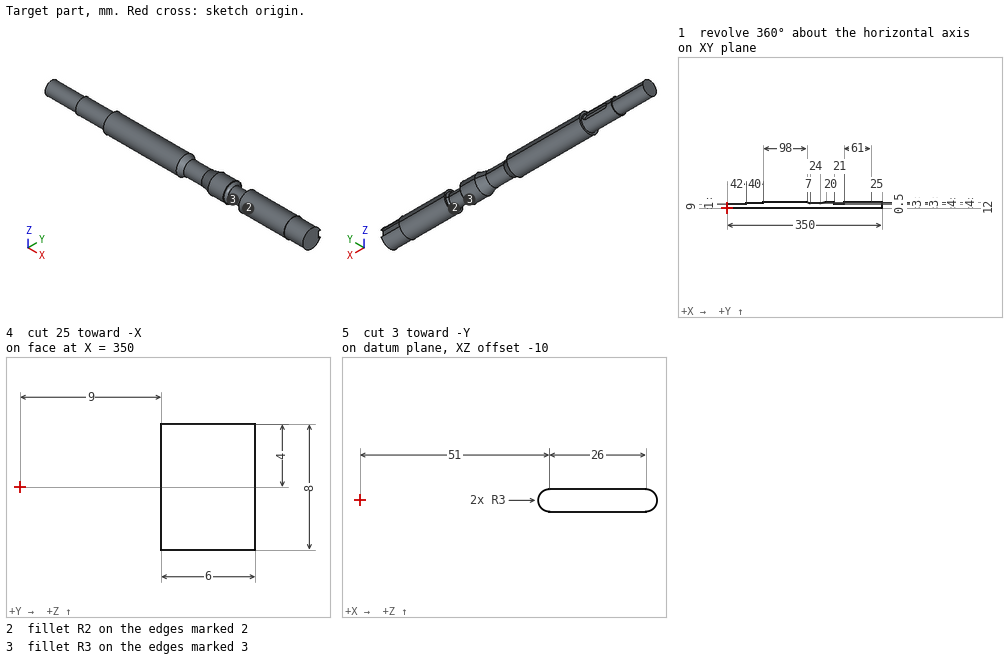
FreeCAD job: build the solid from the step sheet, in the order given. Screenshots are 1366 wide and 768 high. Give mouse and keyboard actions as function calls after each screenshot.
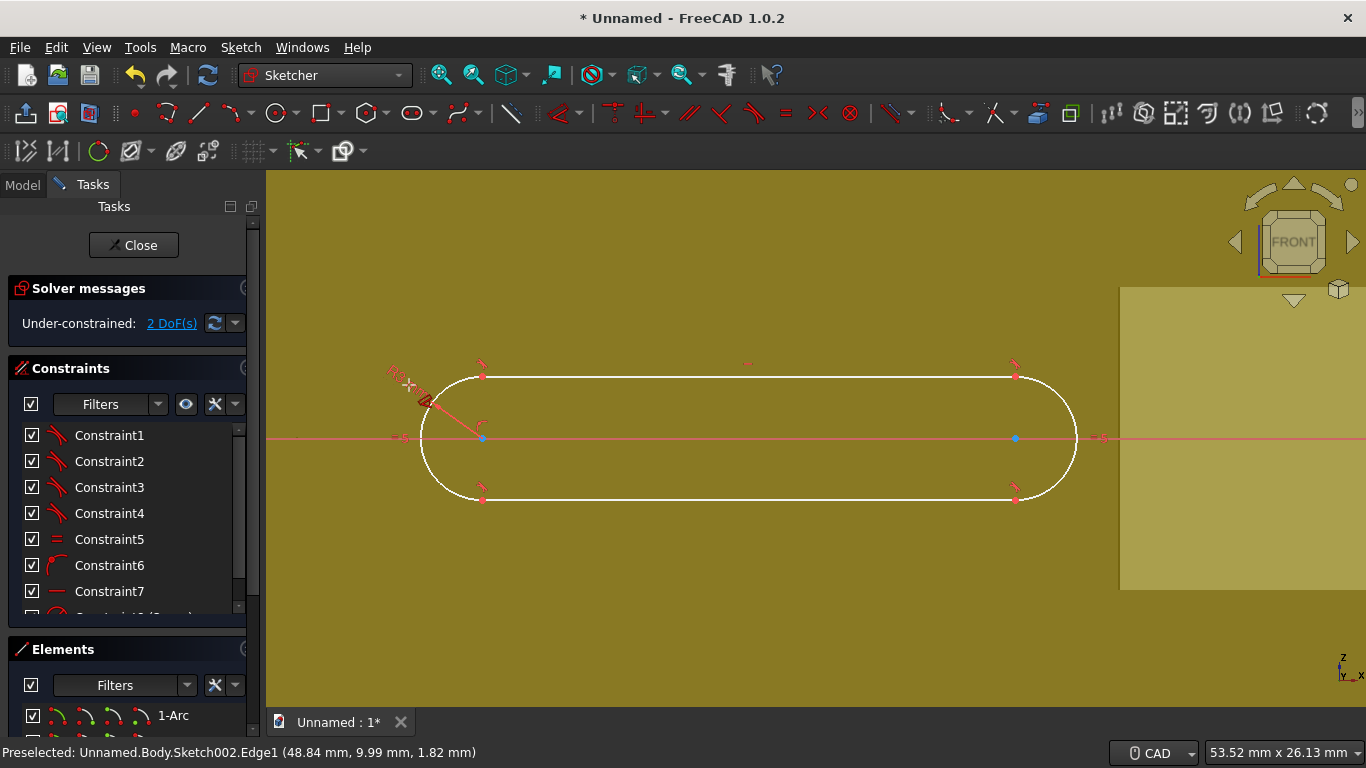
click(642, 377)
click(749, 343)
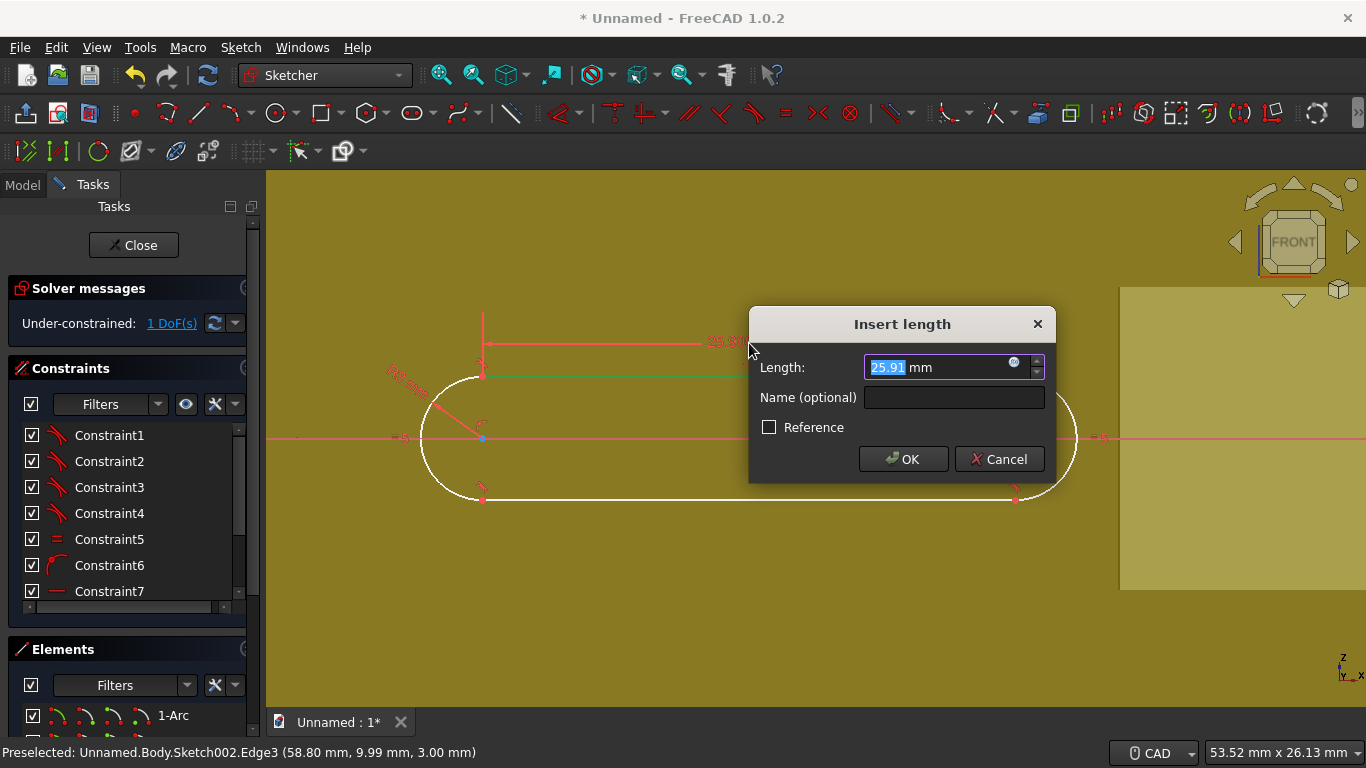
text(26)
key(Return)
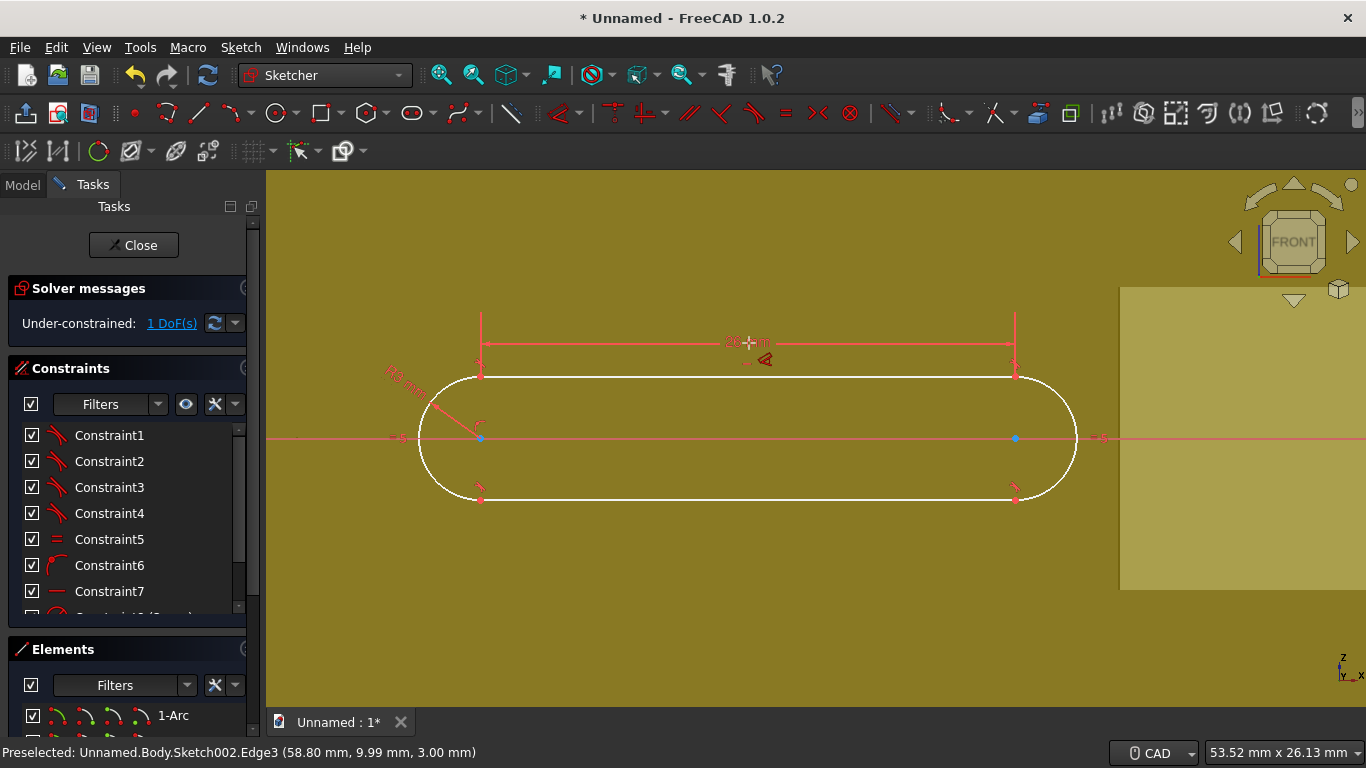
click(481, 377)
click(387, 343)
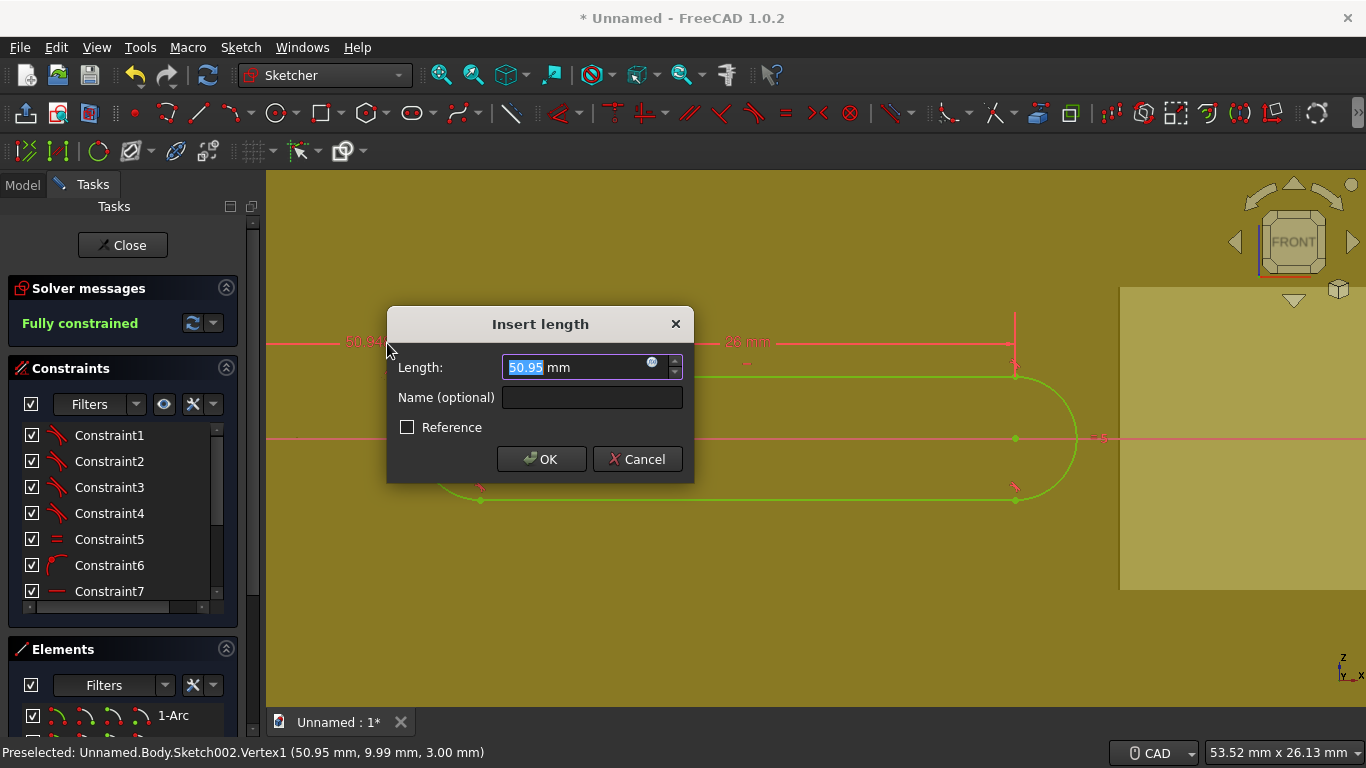
text(51)
key(Return)
key(Escape)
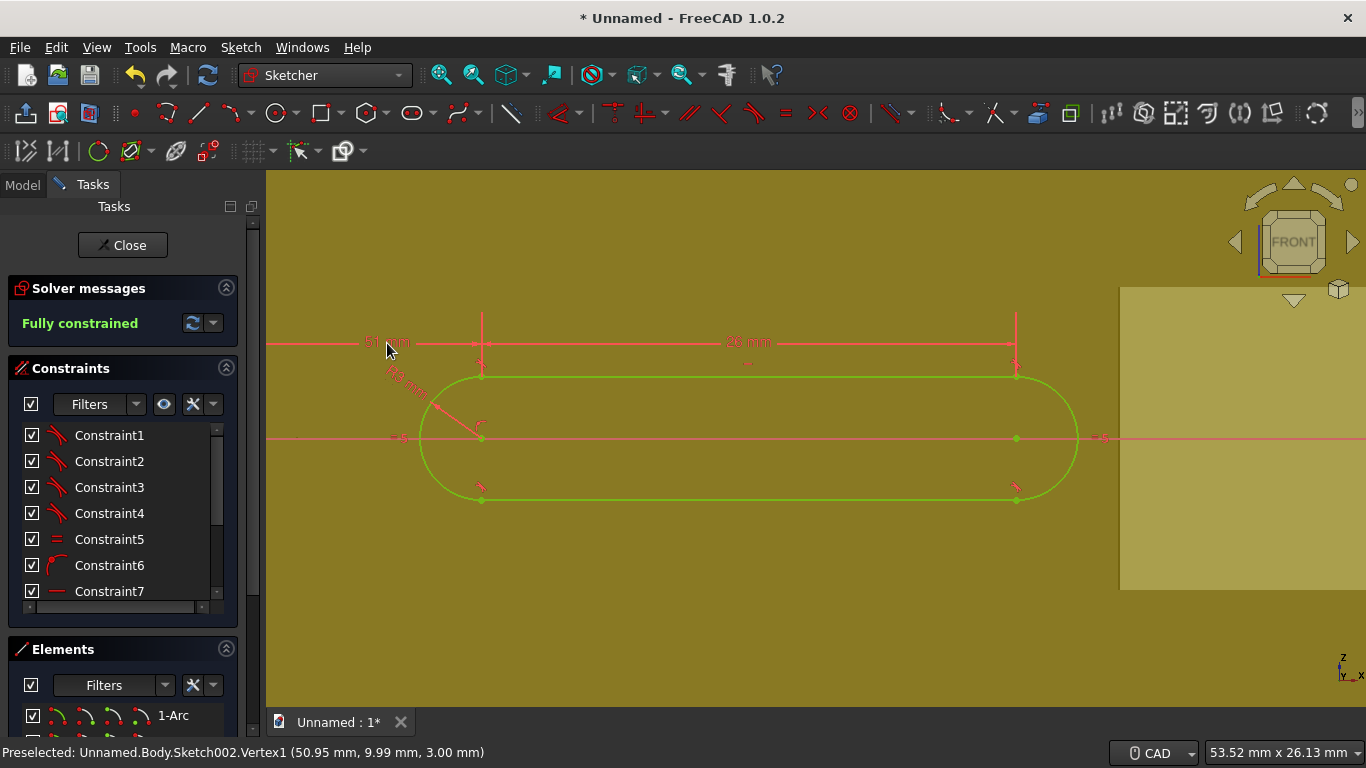
click(123, 245)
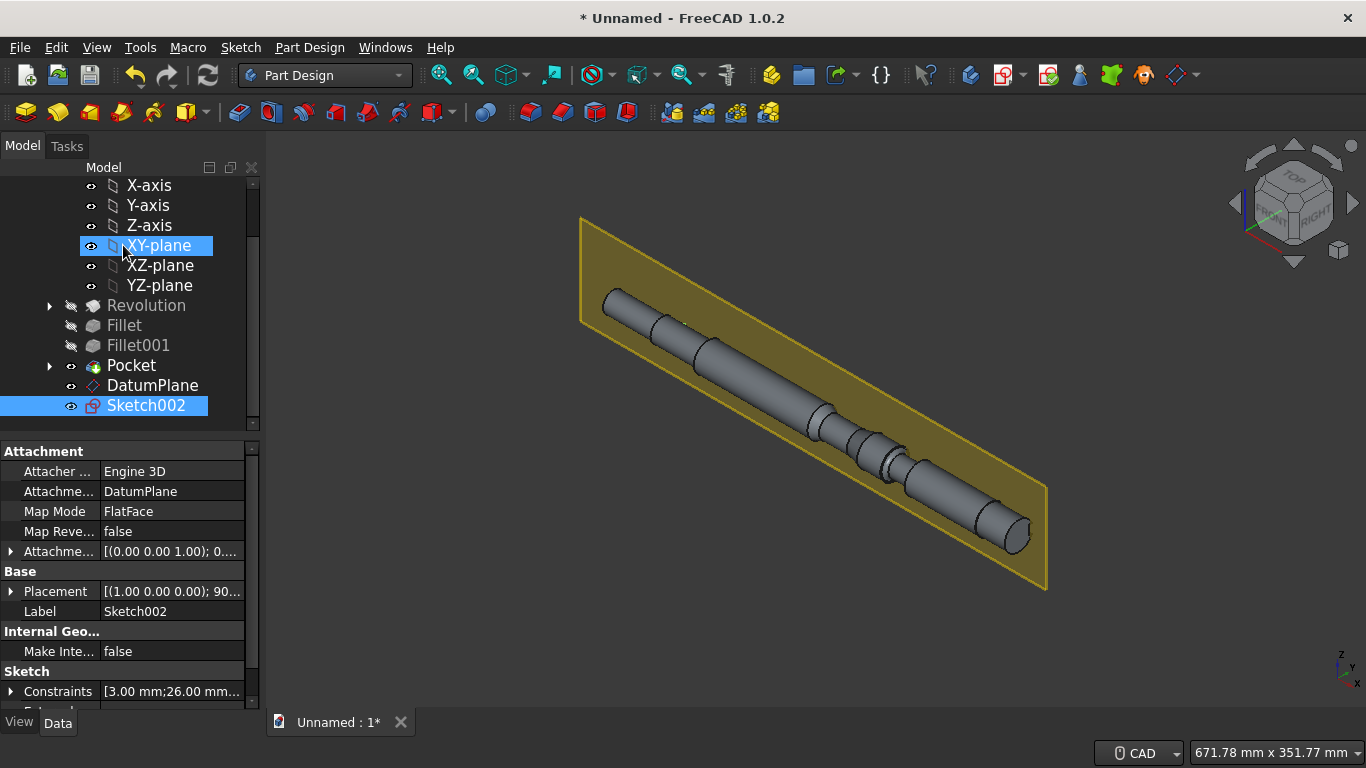
click(240, 112)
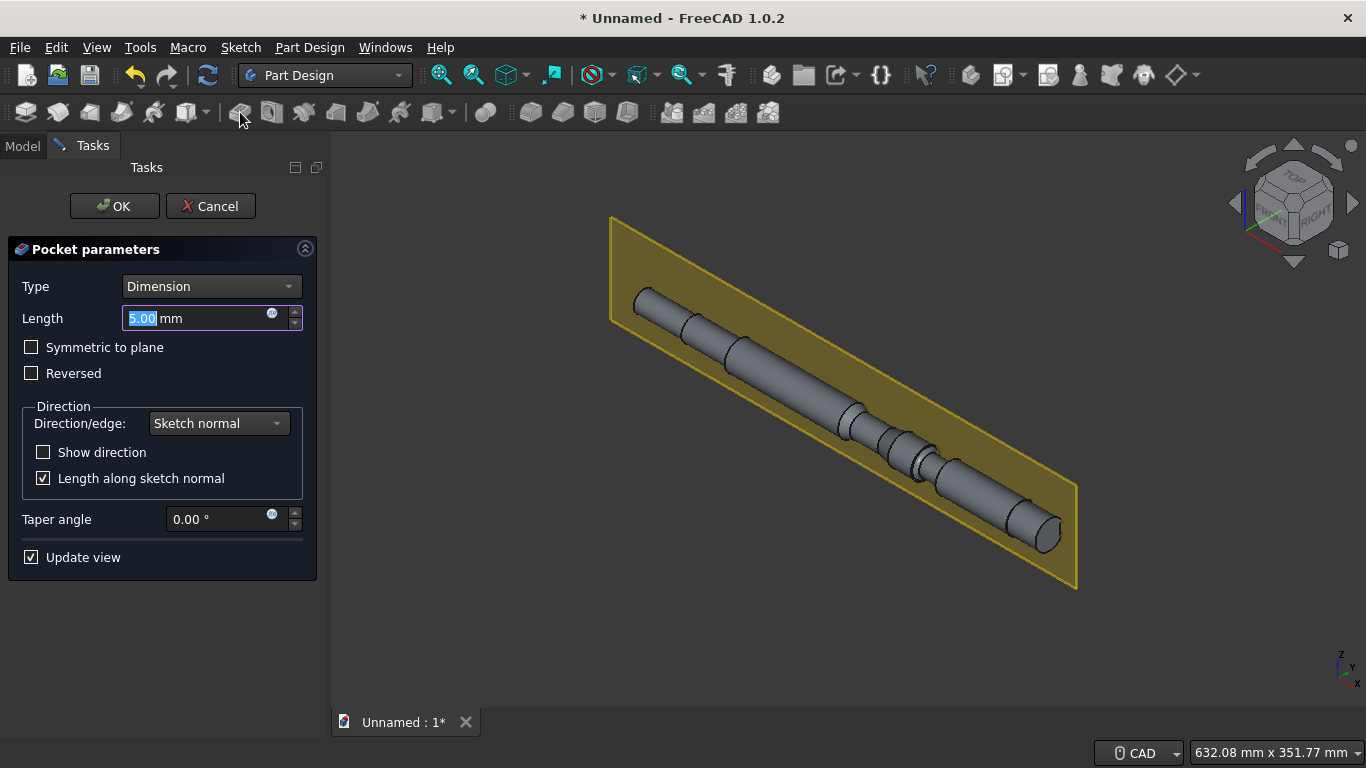
text(3)
key(Tab)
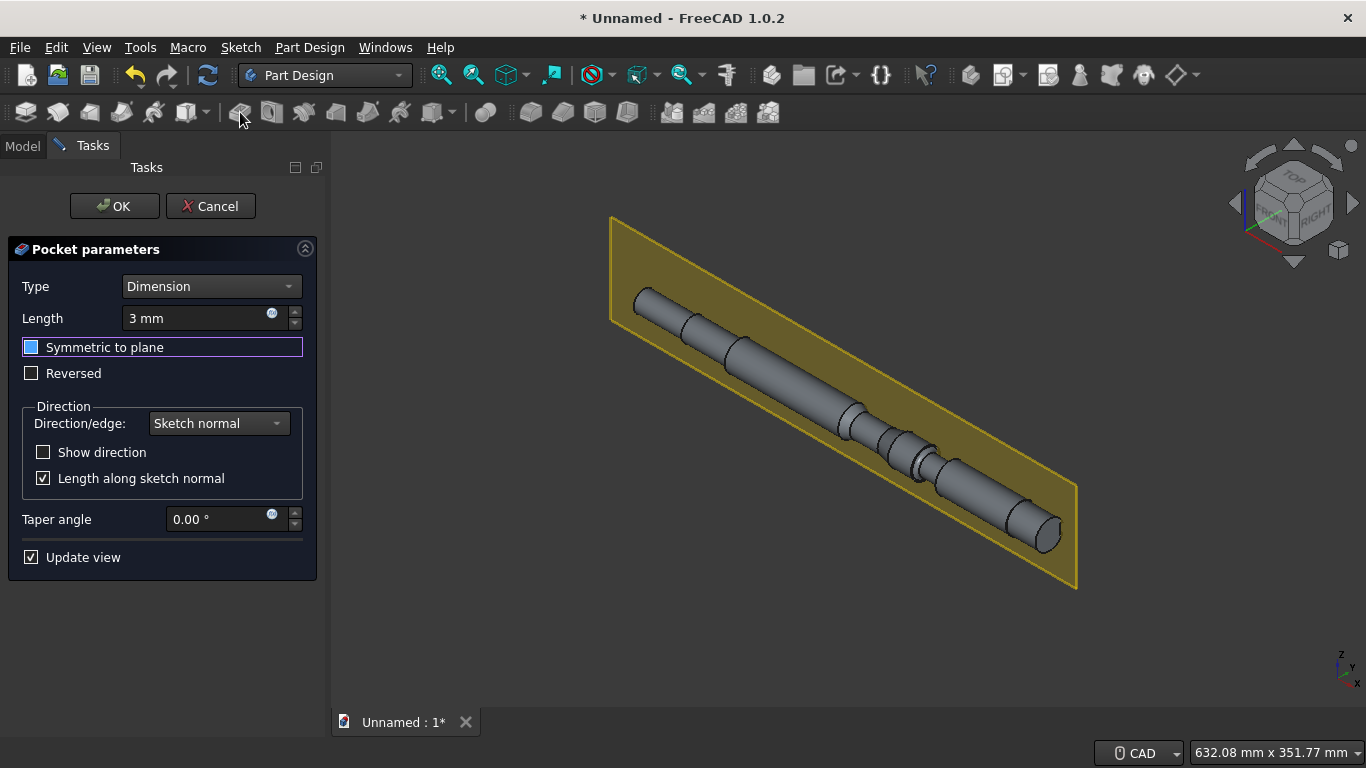
click(30, 373)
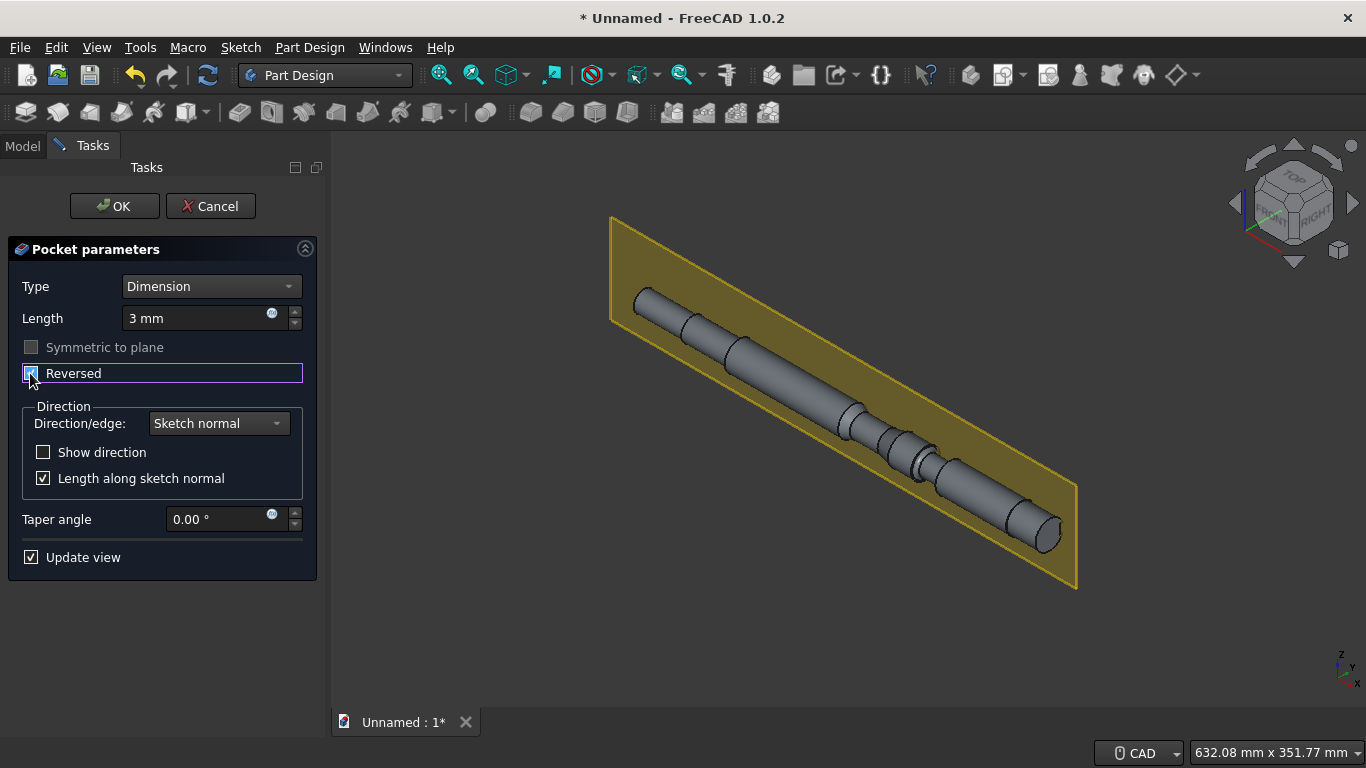
click(115, 206)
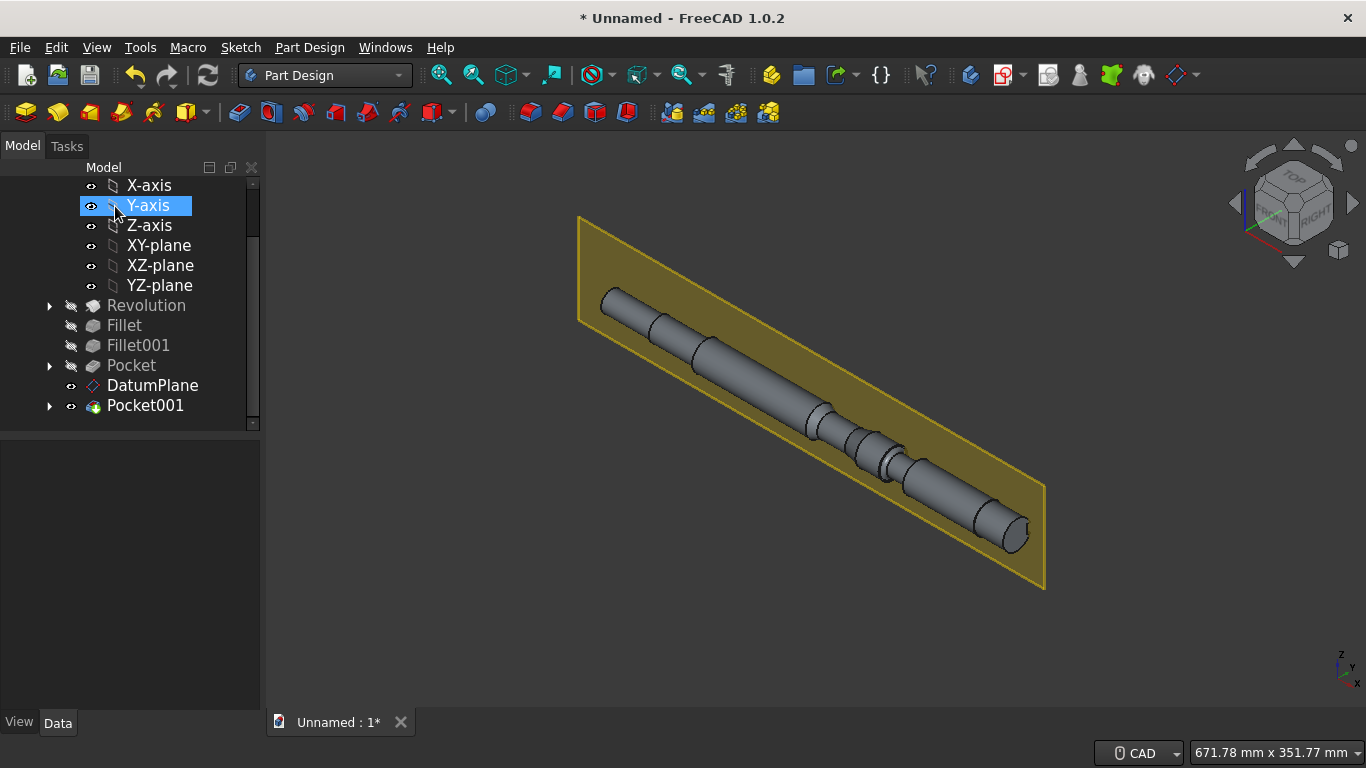
click(116, 386)
key(space)